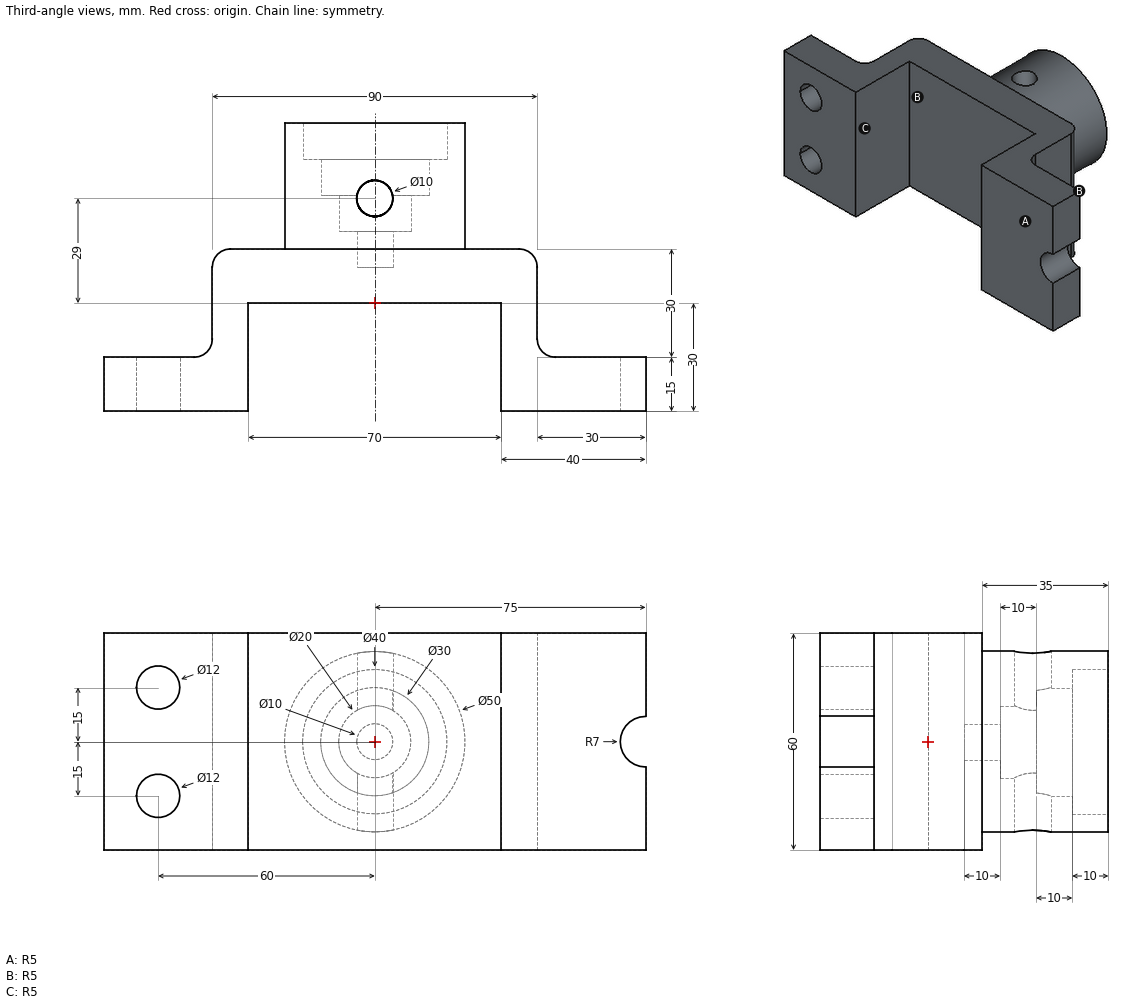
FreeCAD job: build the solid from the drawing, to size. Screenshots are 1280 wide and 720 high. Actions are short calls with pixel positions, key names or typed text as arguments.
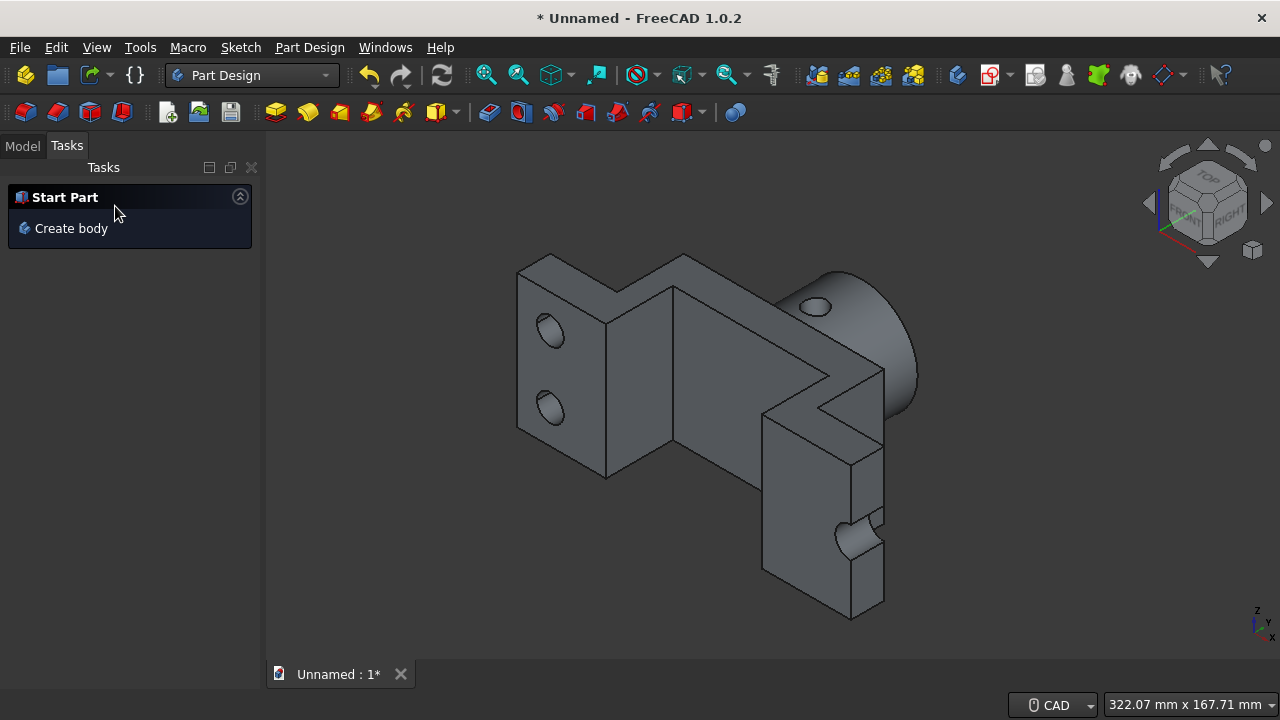
key(1)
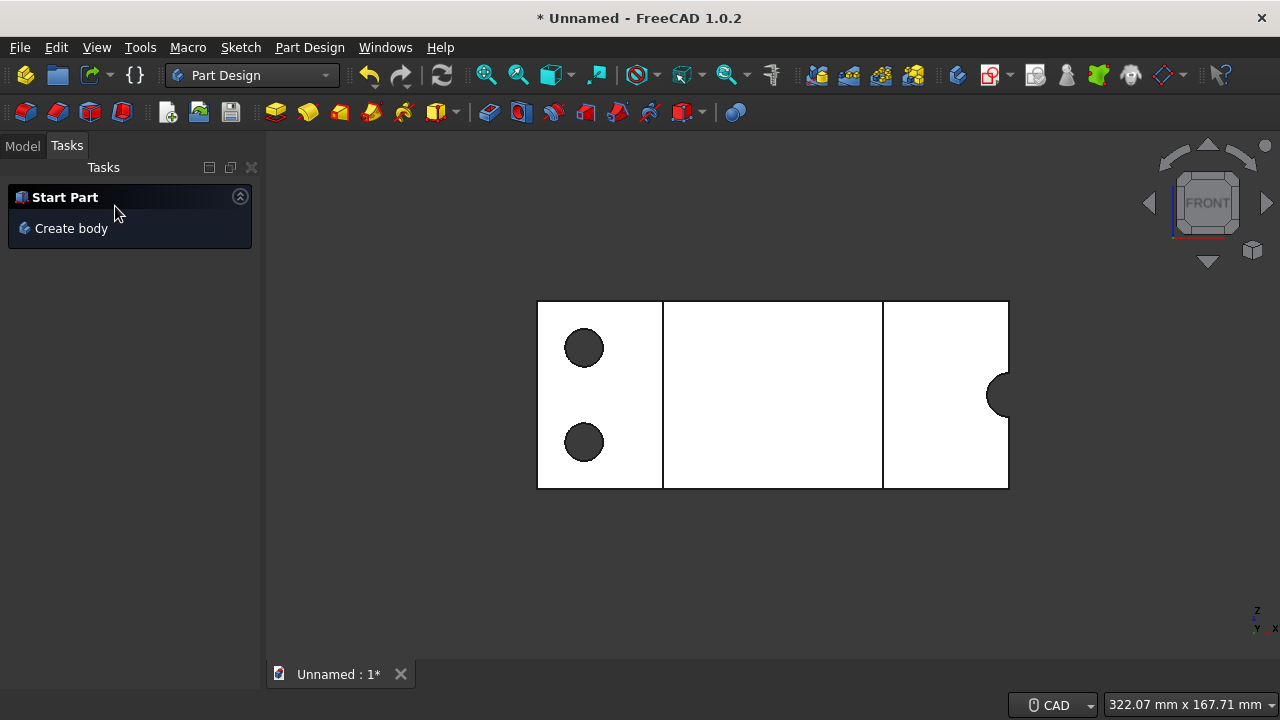
key(3)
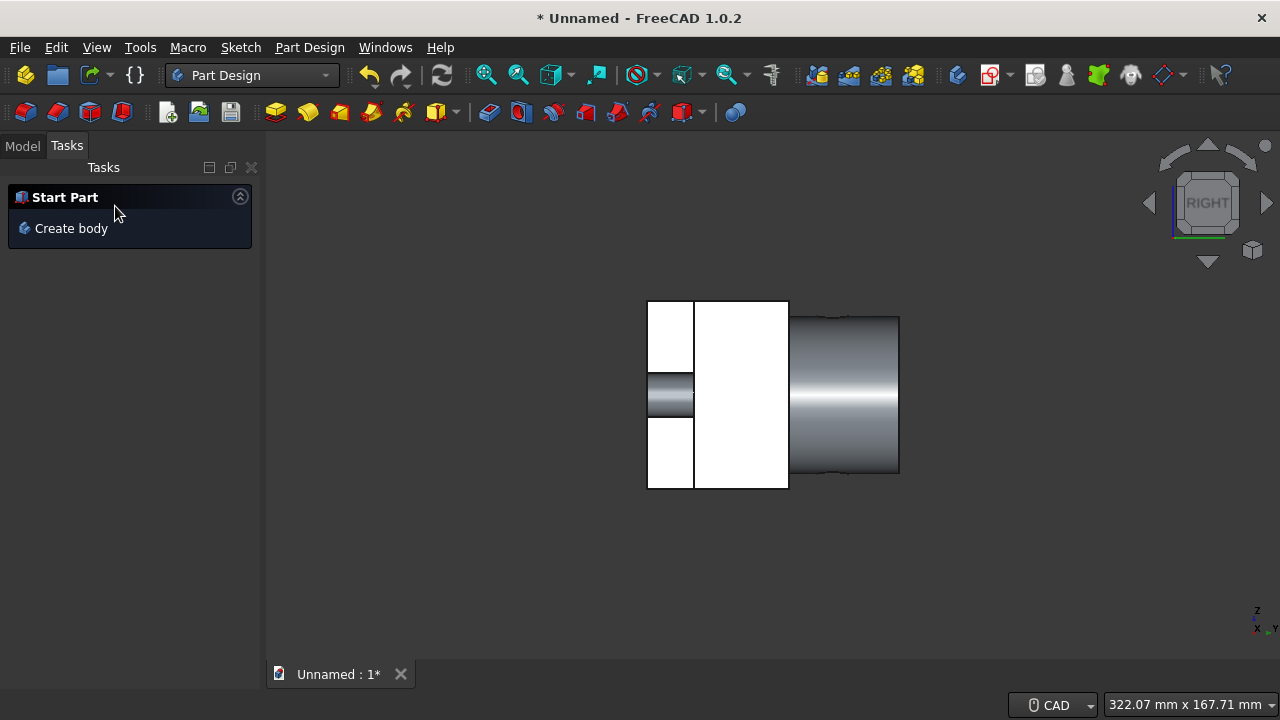
click(488, 76)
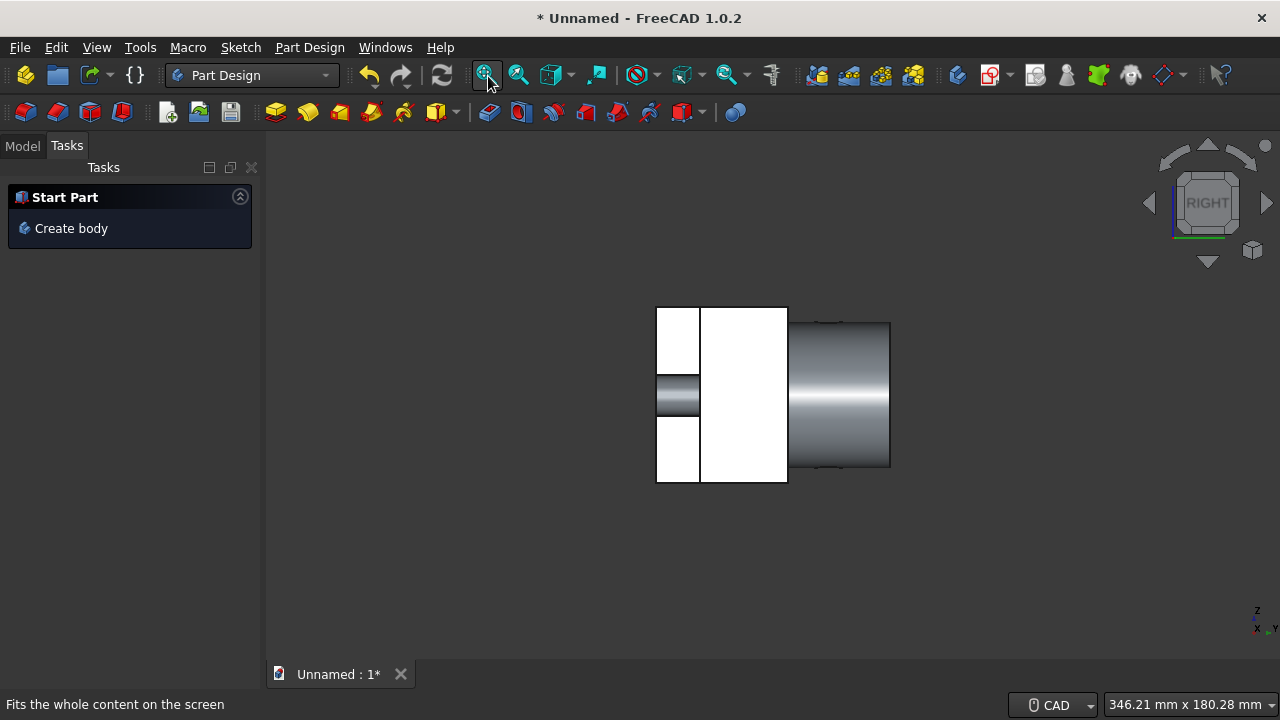
key(5)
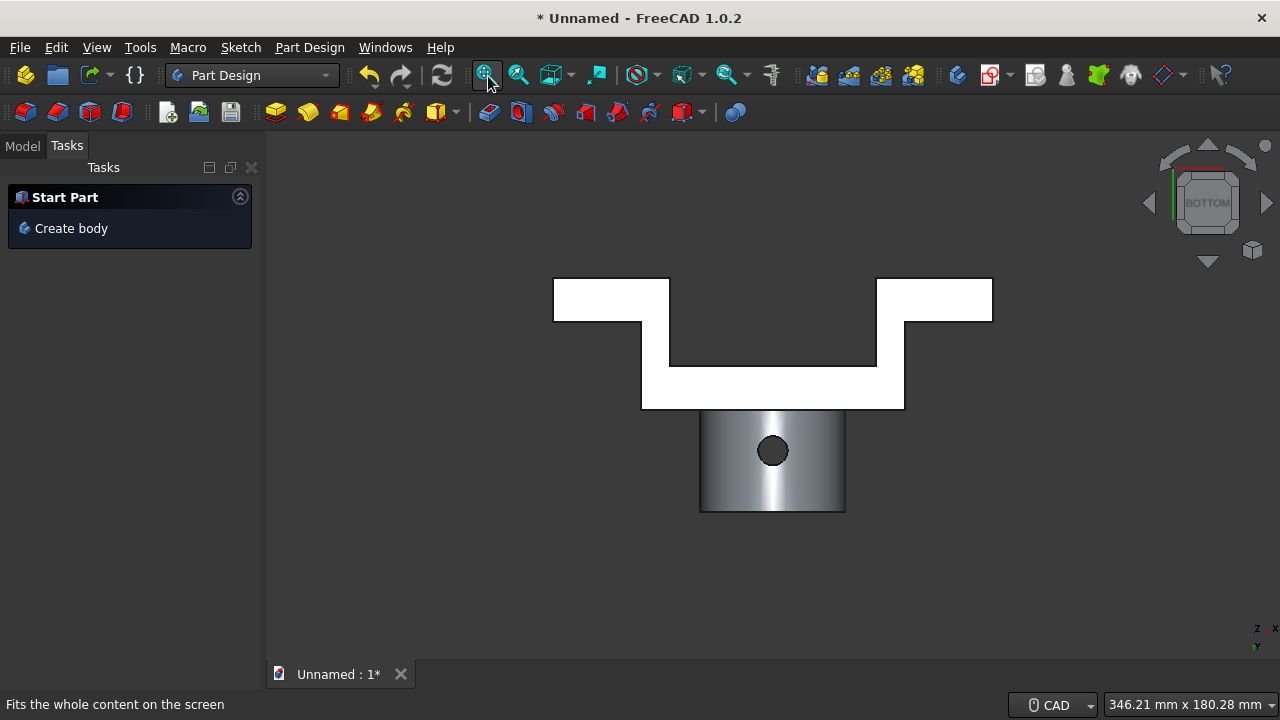
key(v)
key(f)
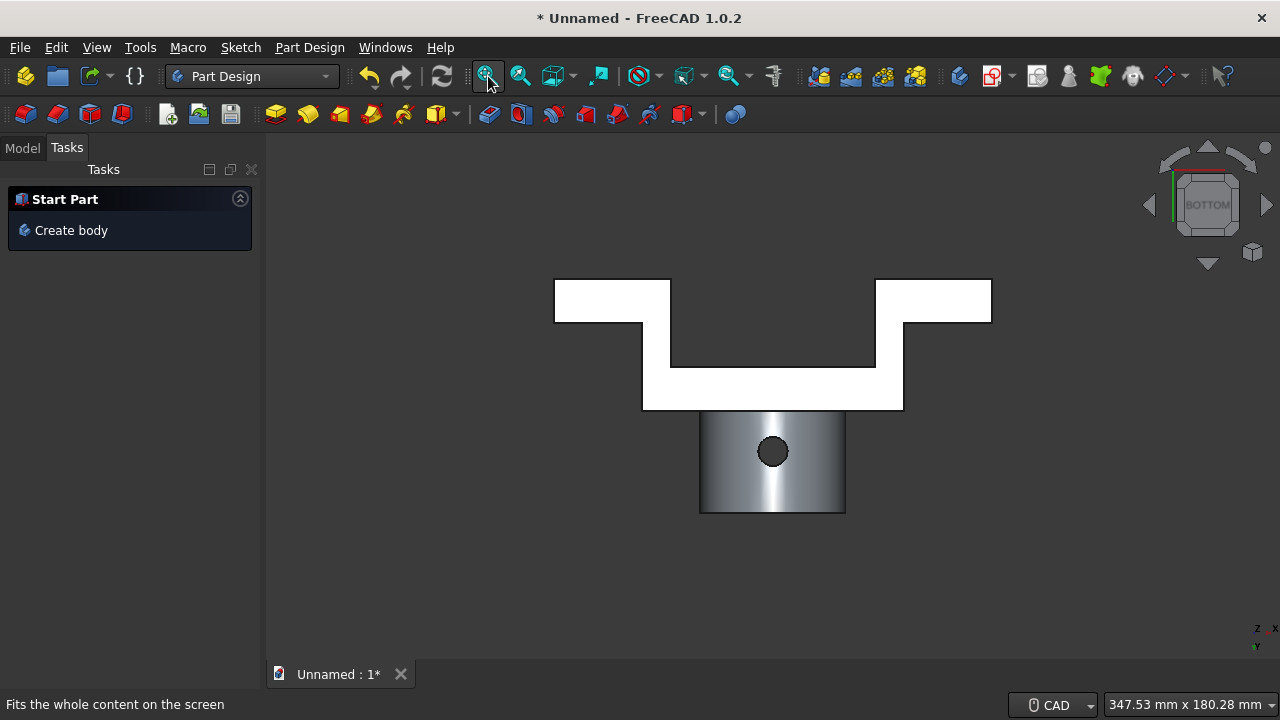
key(4)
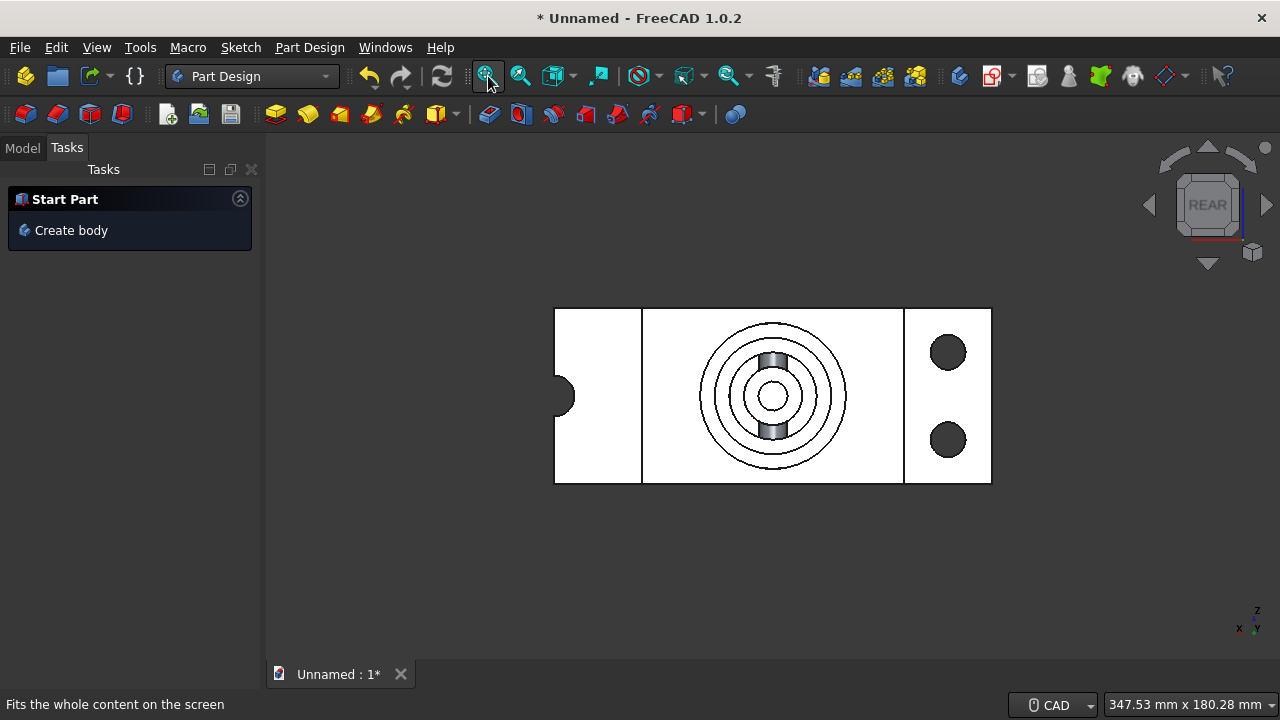
click(488, 76)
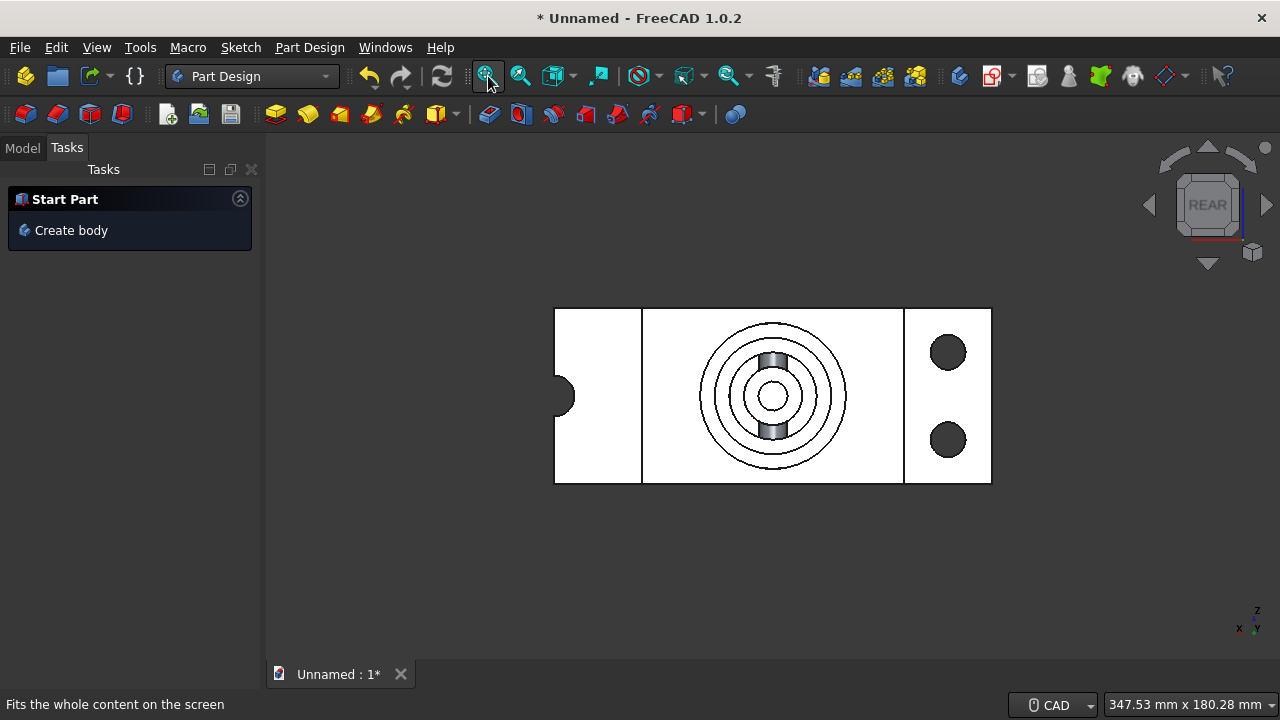
key(6)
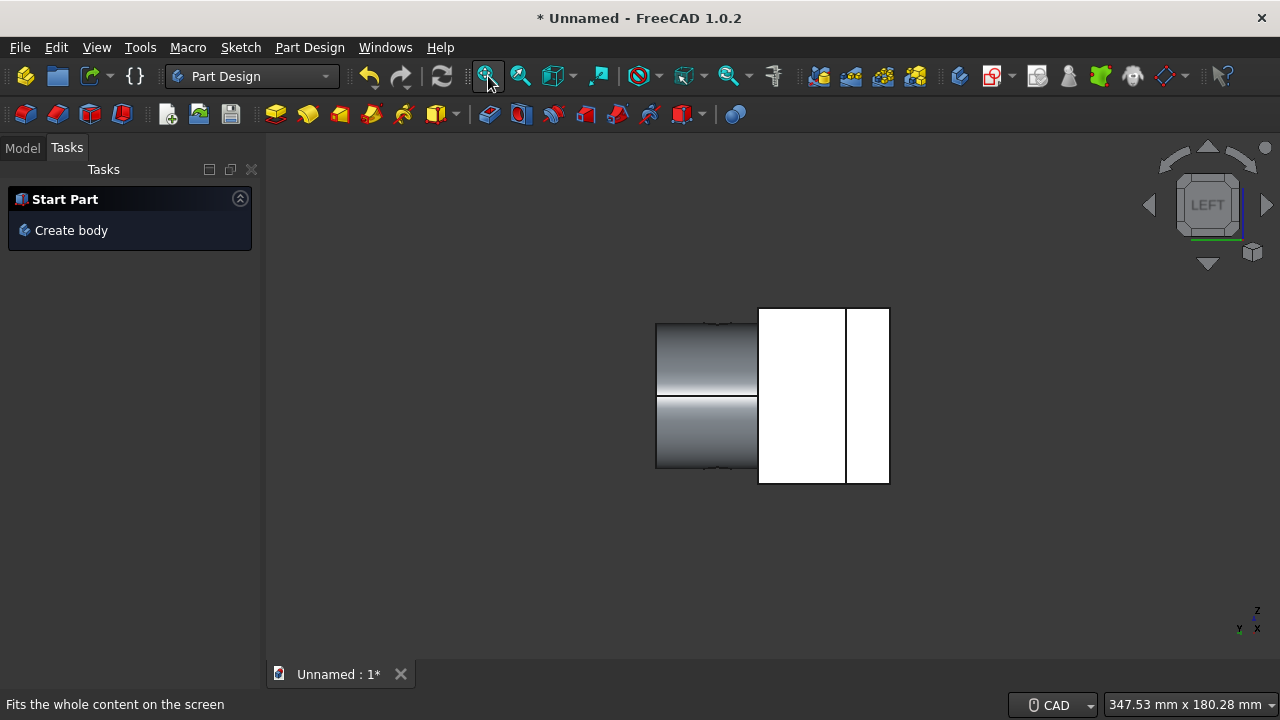
key(v)
key(f)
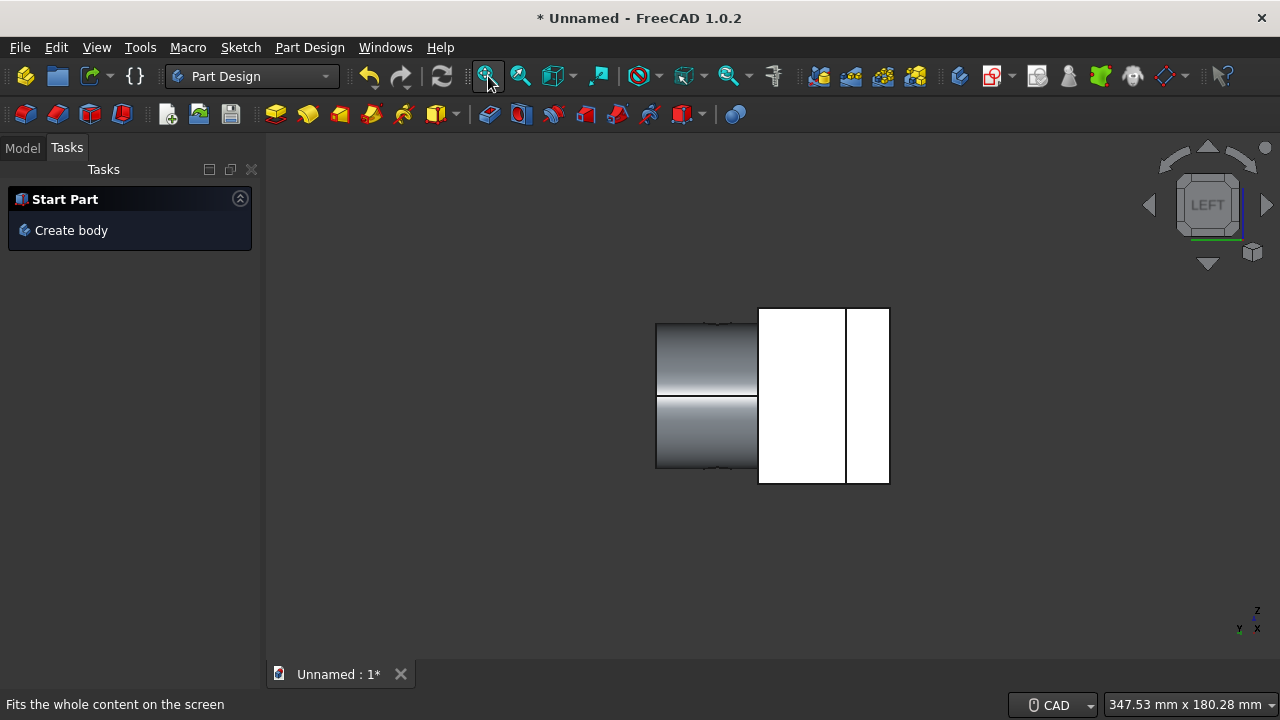
key(v)
key(3)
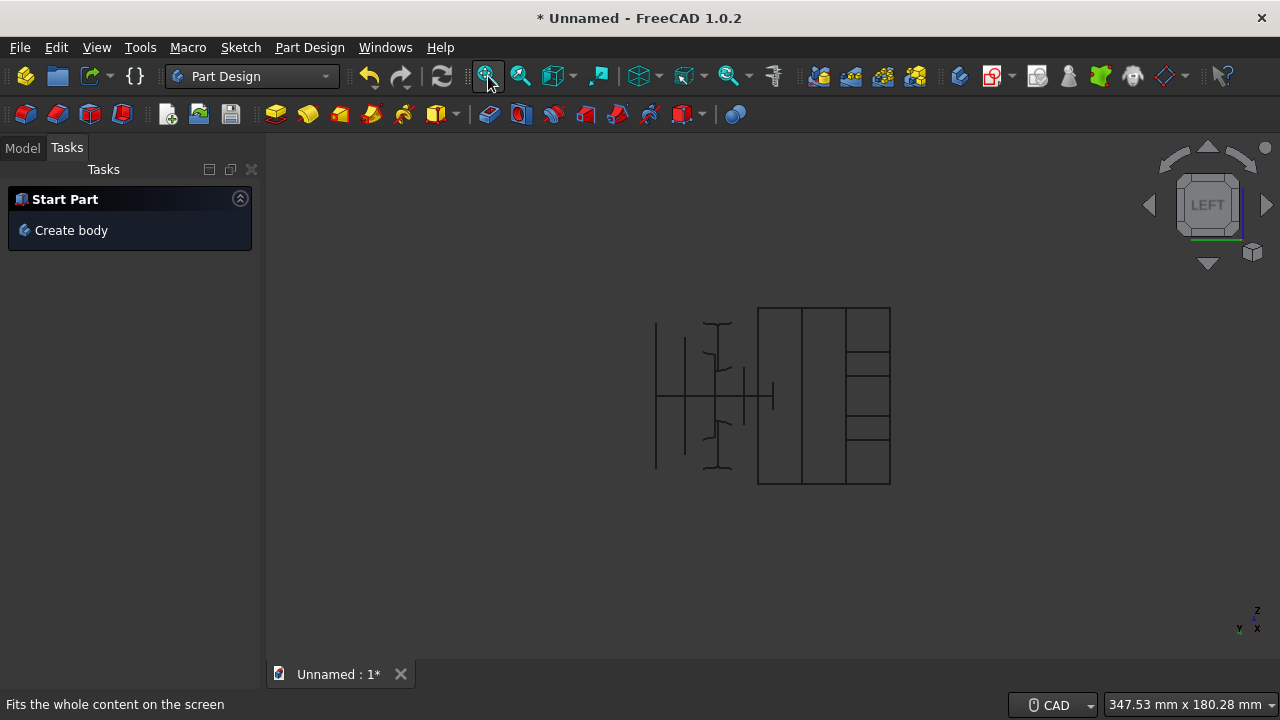
key(0)